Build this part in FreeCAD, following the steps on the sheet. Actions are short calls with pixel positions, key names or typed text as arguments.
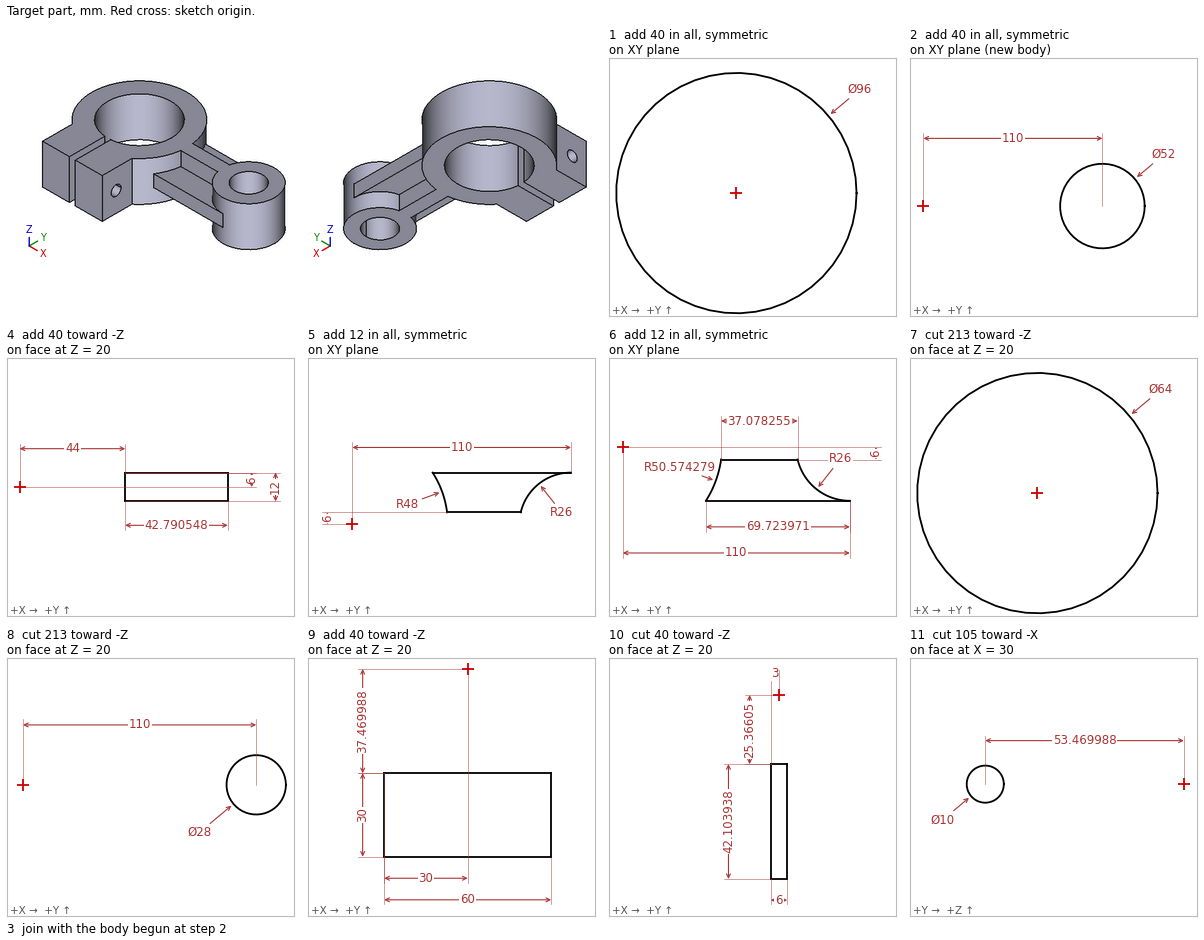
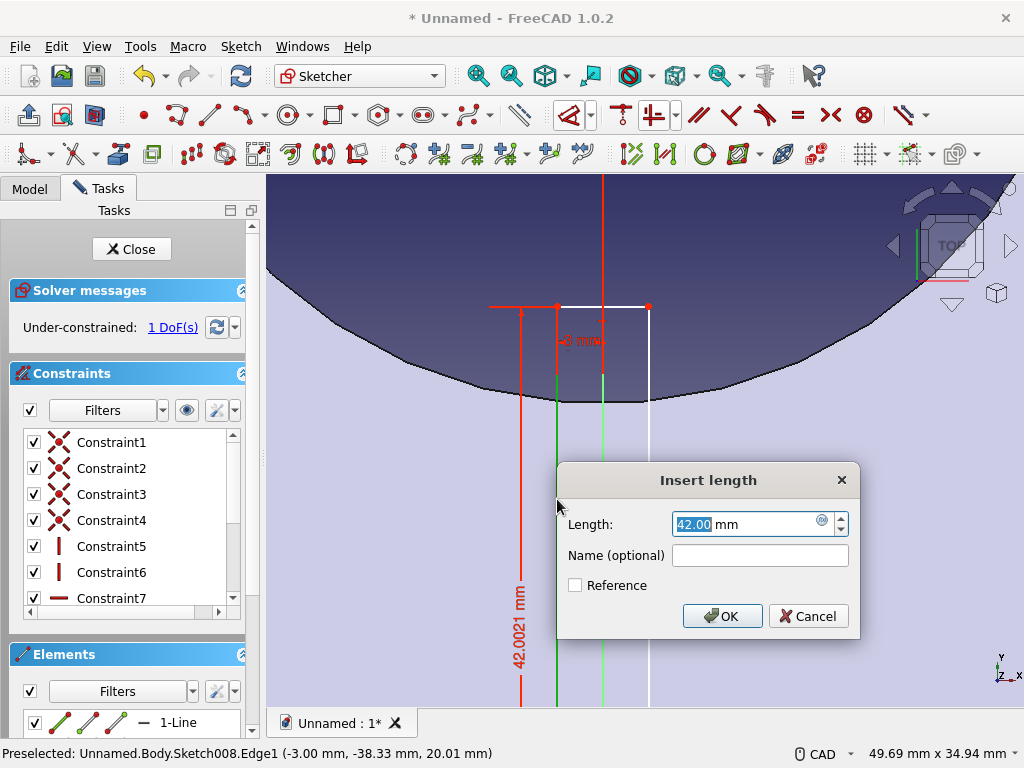
text(42.103938)
key(Return)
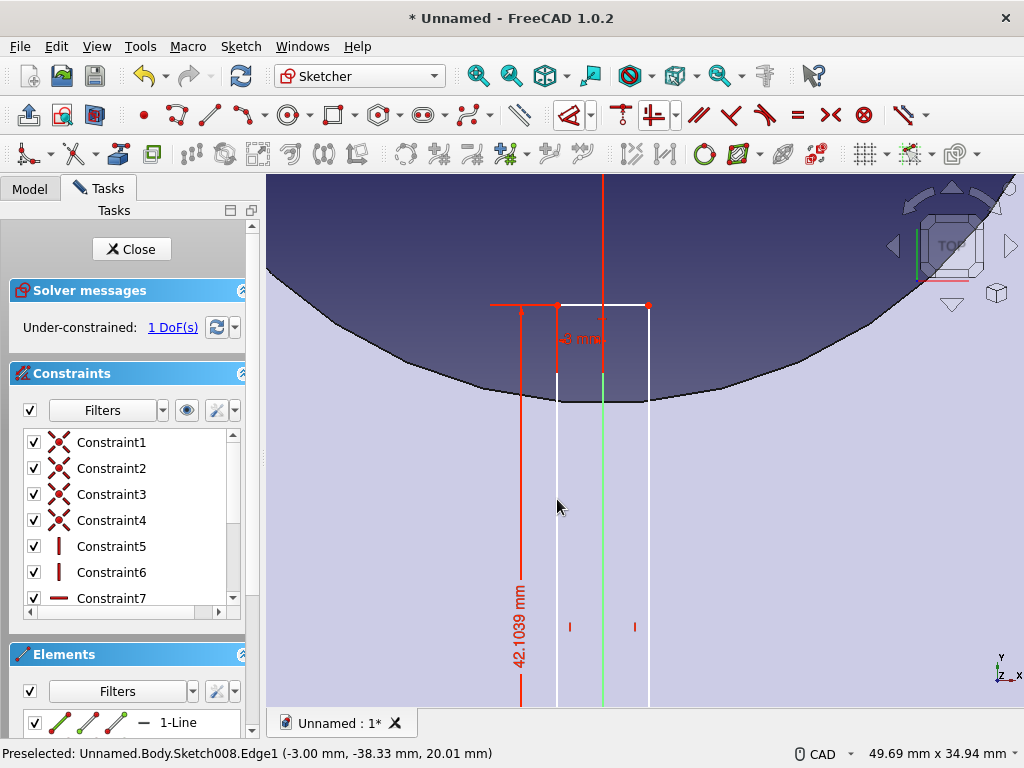
click(557, 305)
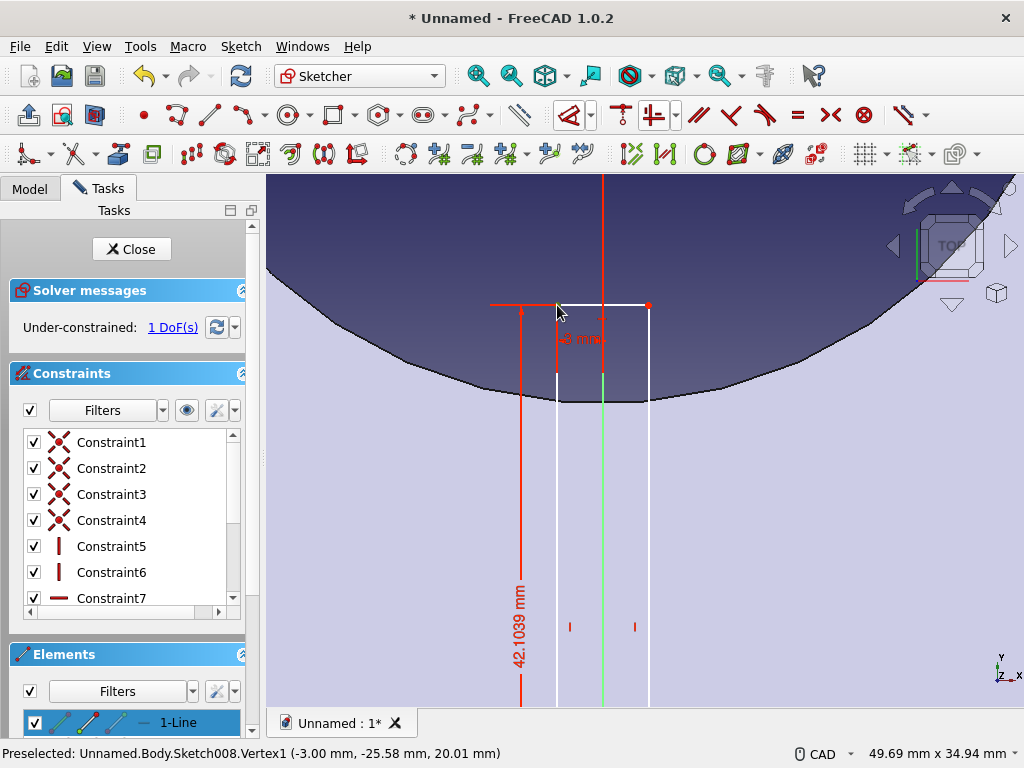
click(590, 116)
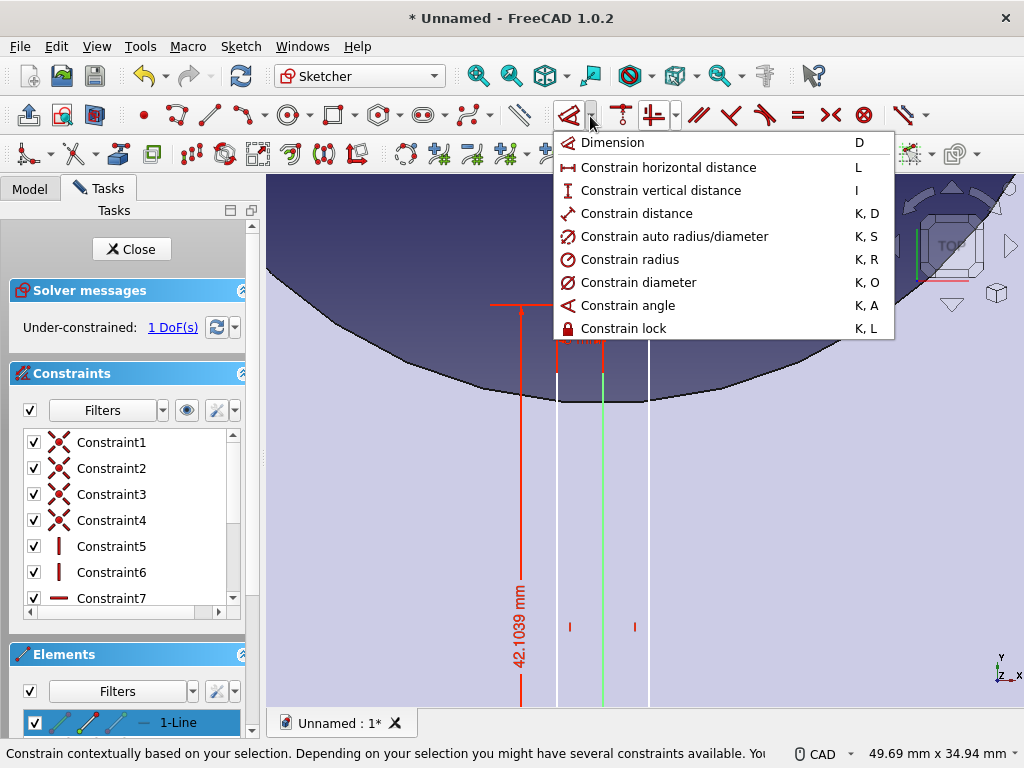
click(724, 190)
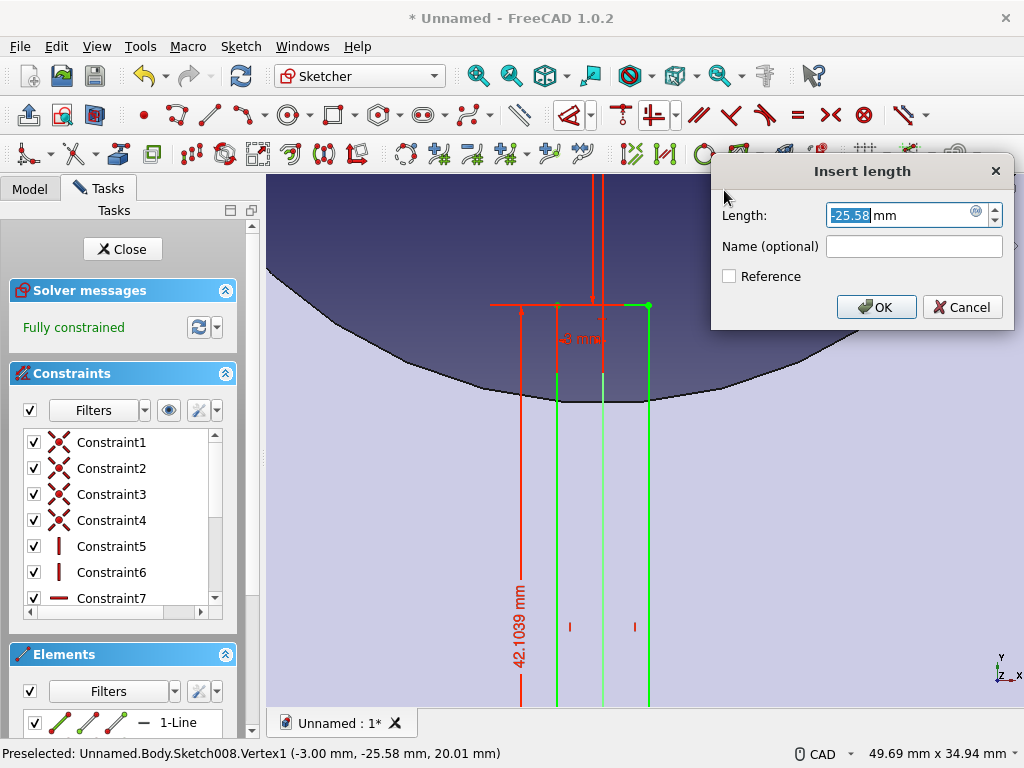
text(-25.36605)
key(Return)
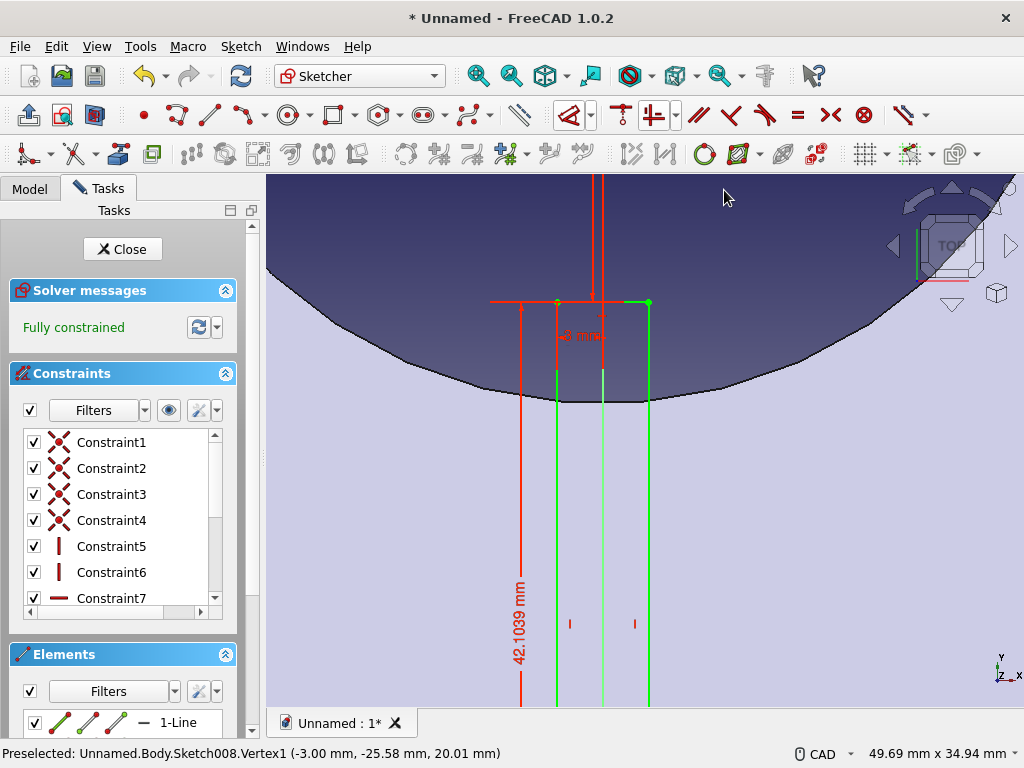
click(123, 249)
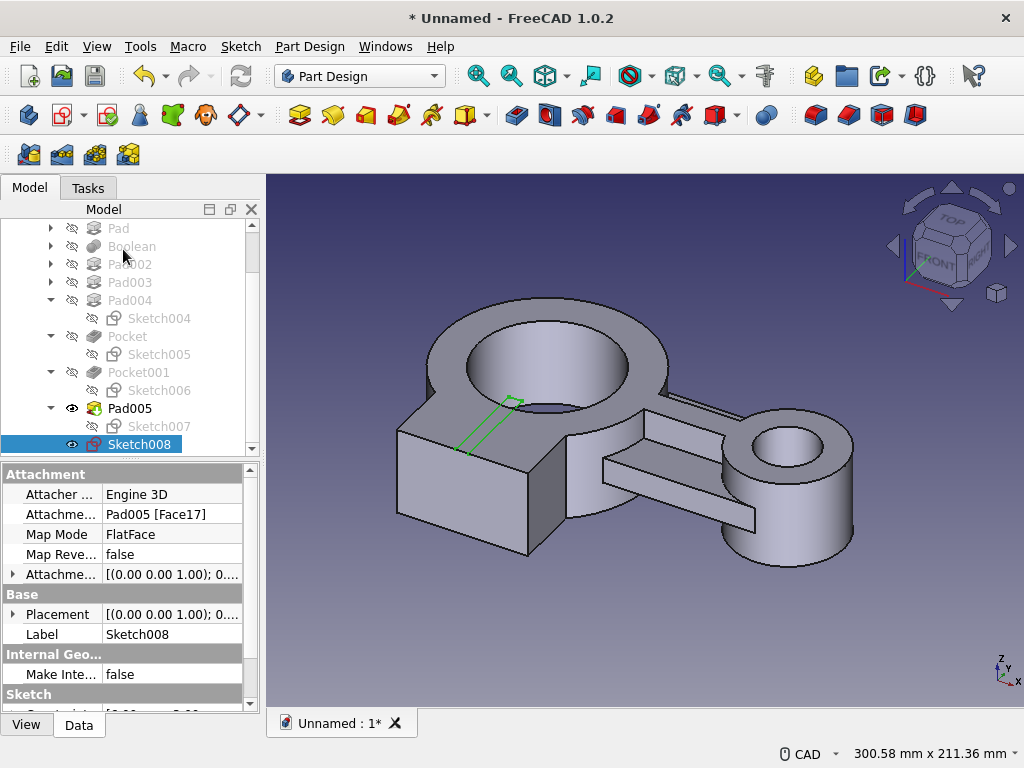
click(517, 116)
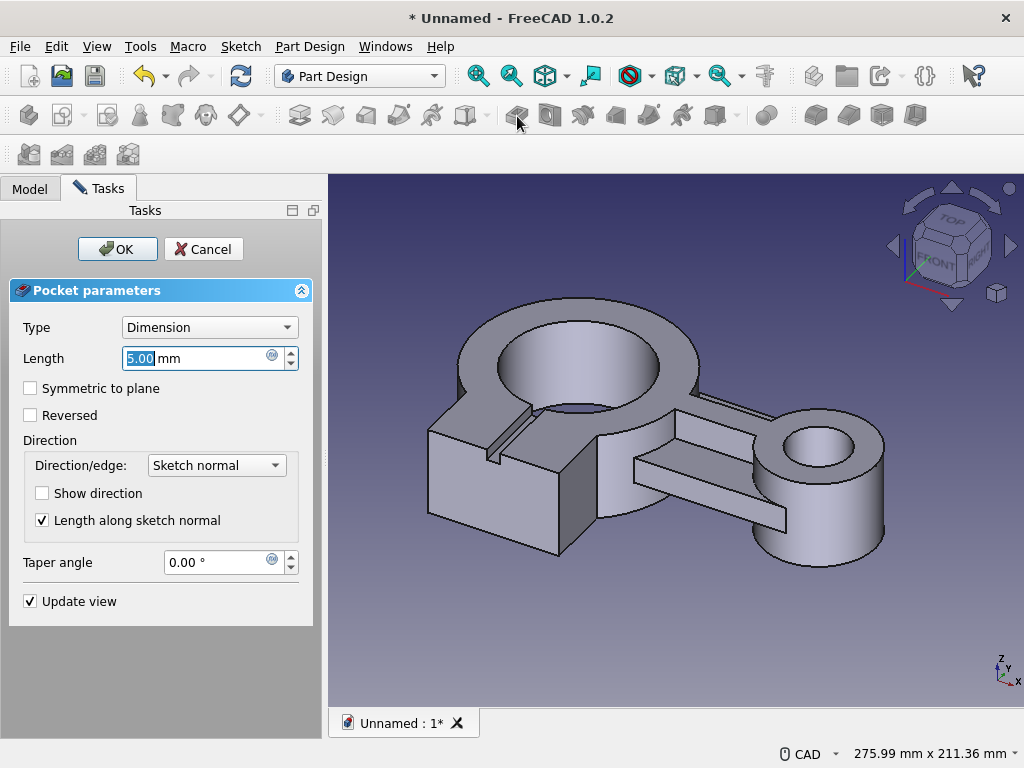
text(40)
key(Tab)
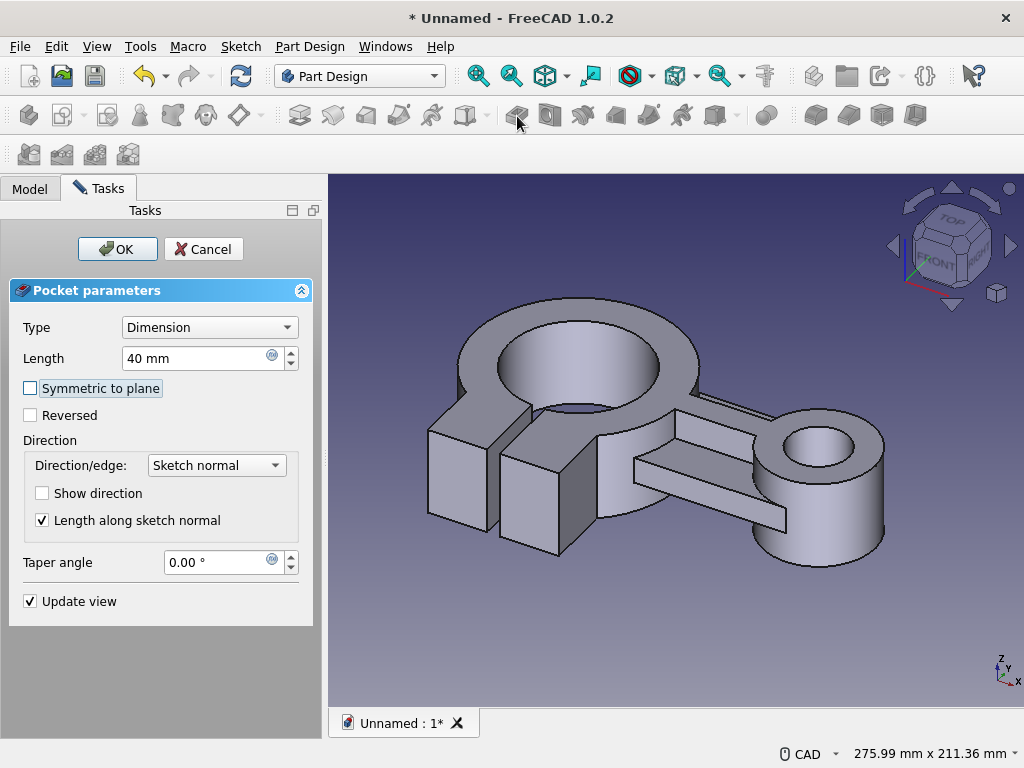
click(118, 249)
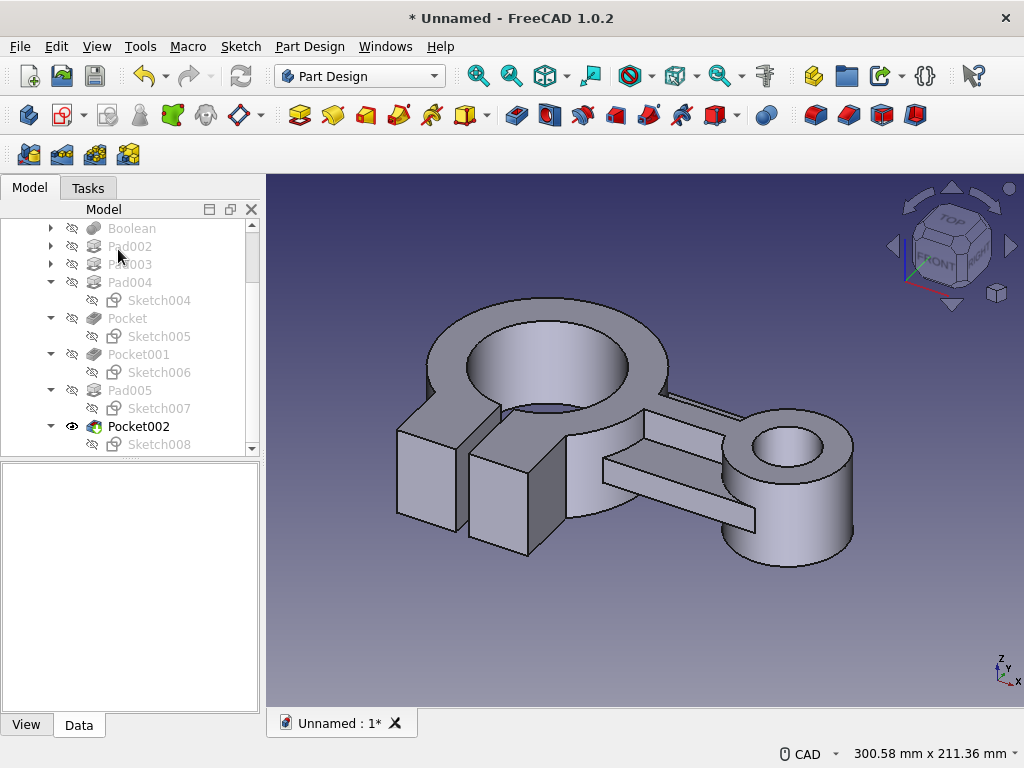
click(547, 495)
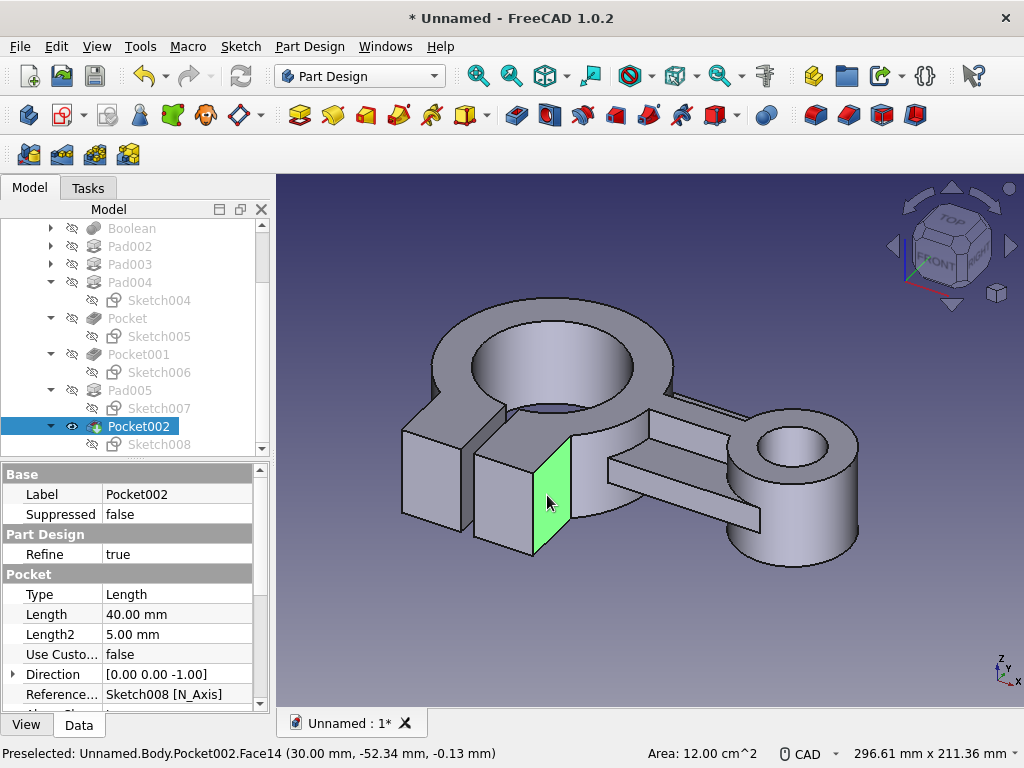
click(62, 116)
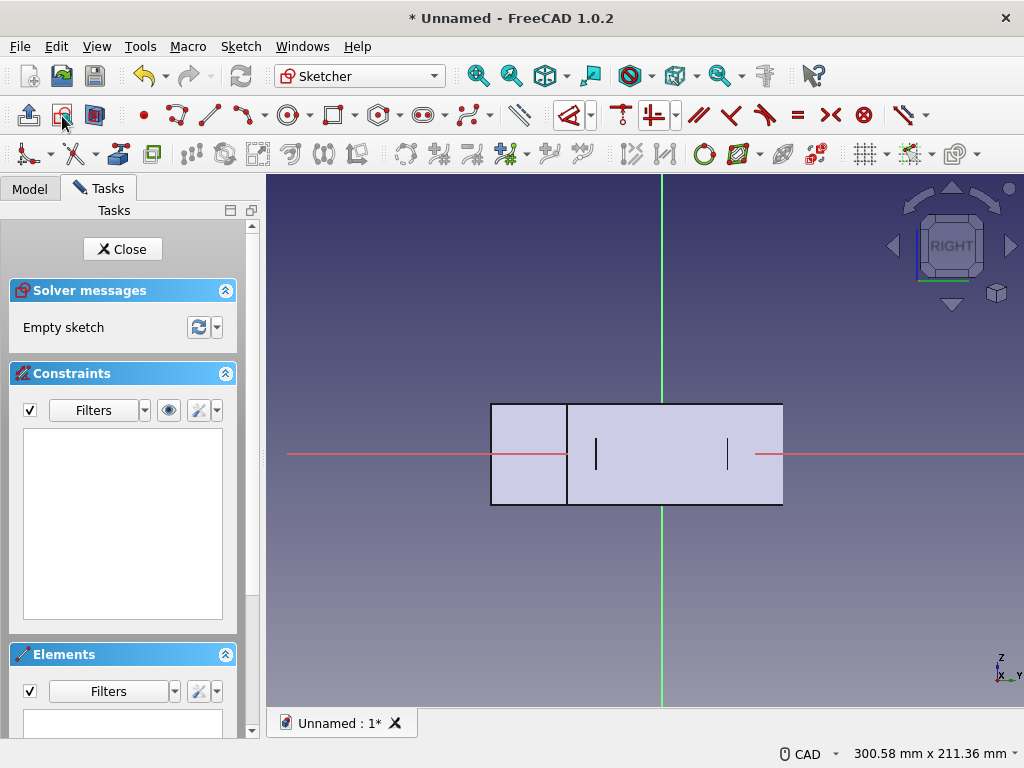
scroll(523, 455, up, 13)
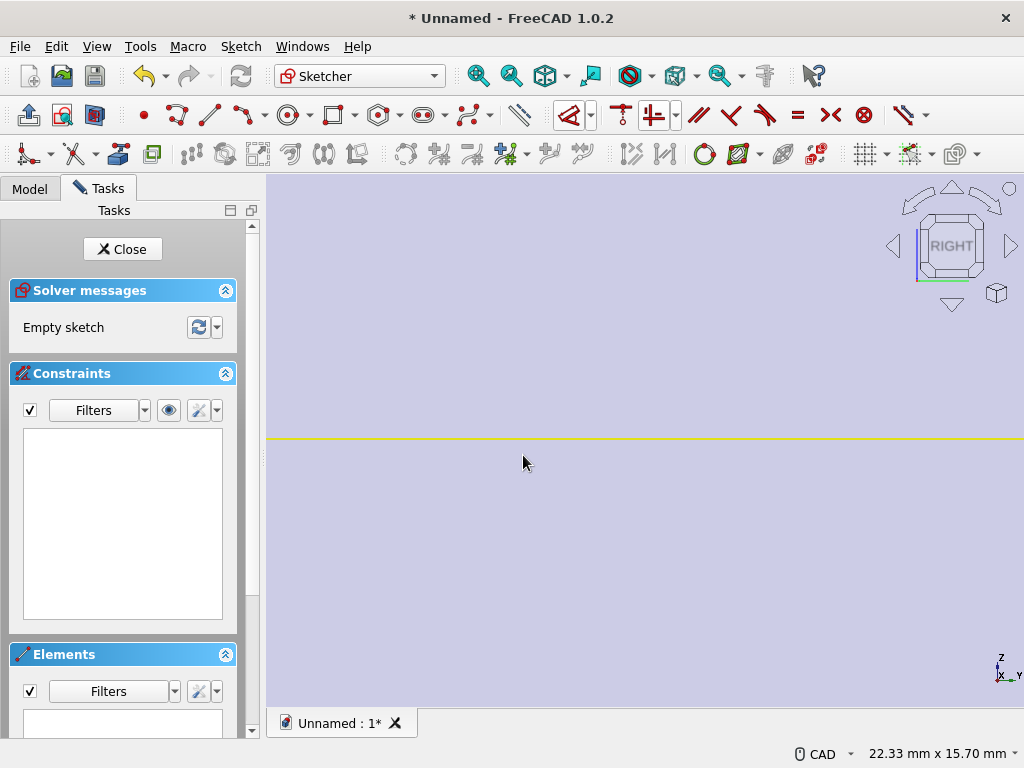
click(288, 116)